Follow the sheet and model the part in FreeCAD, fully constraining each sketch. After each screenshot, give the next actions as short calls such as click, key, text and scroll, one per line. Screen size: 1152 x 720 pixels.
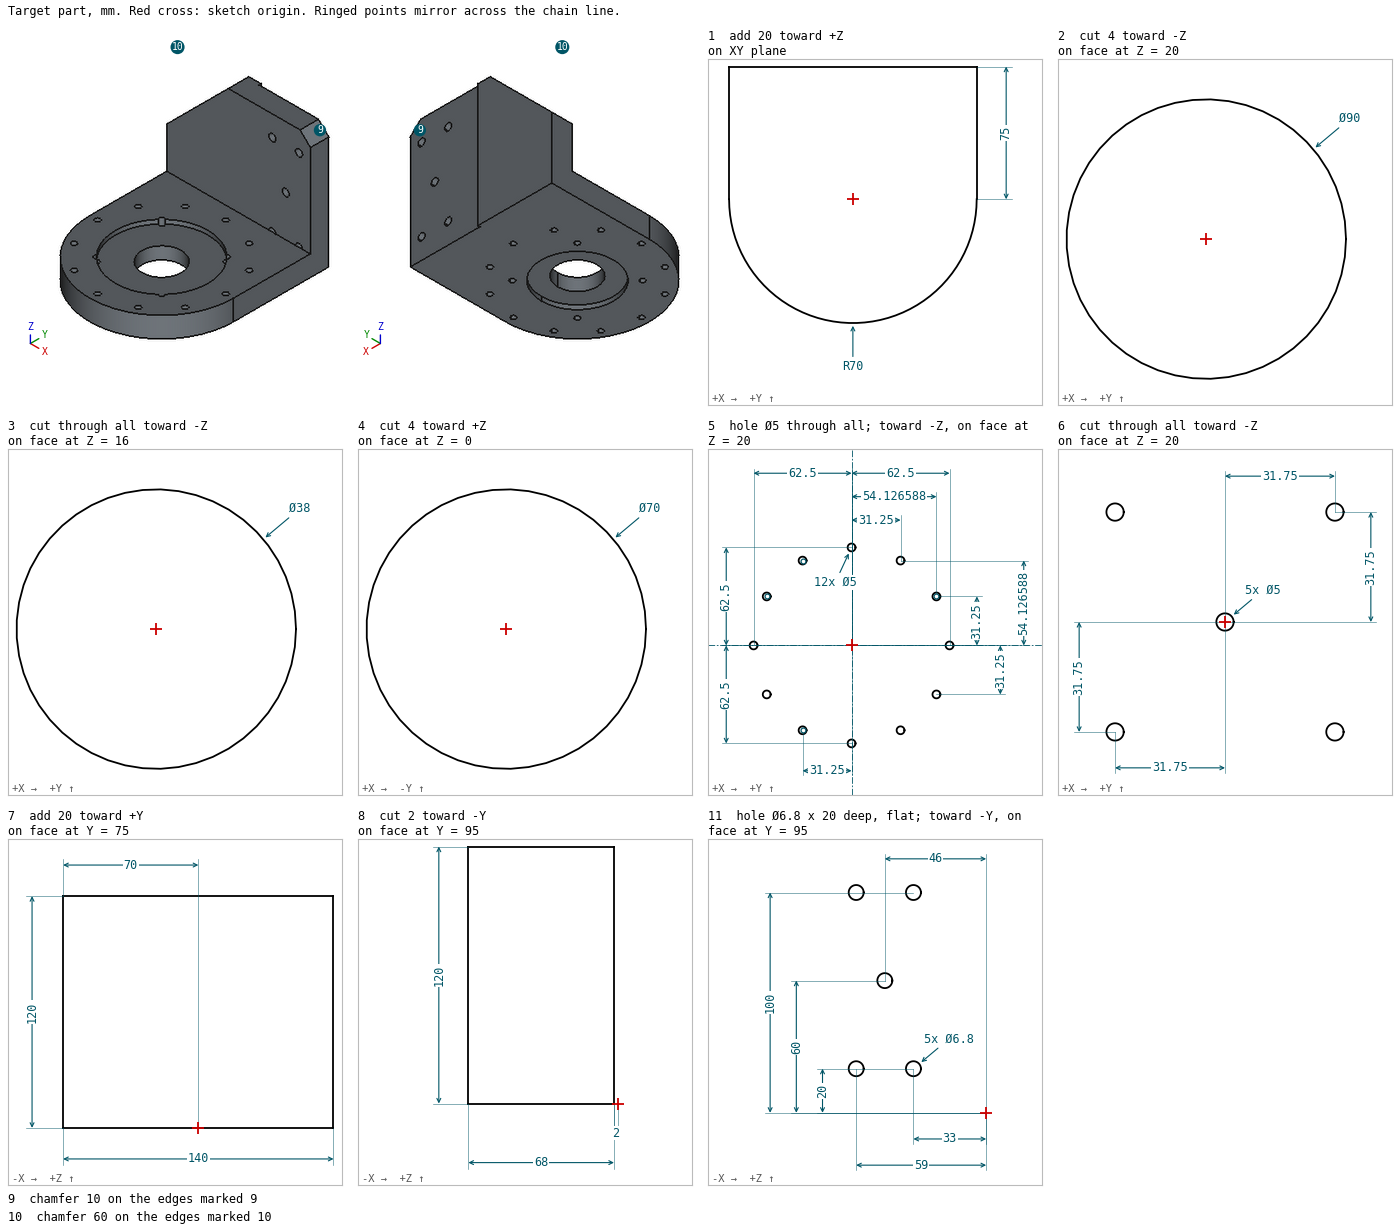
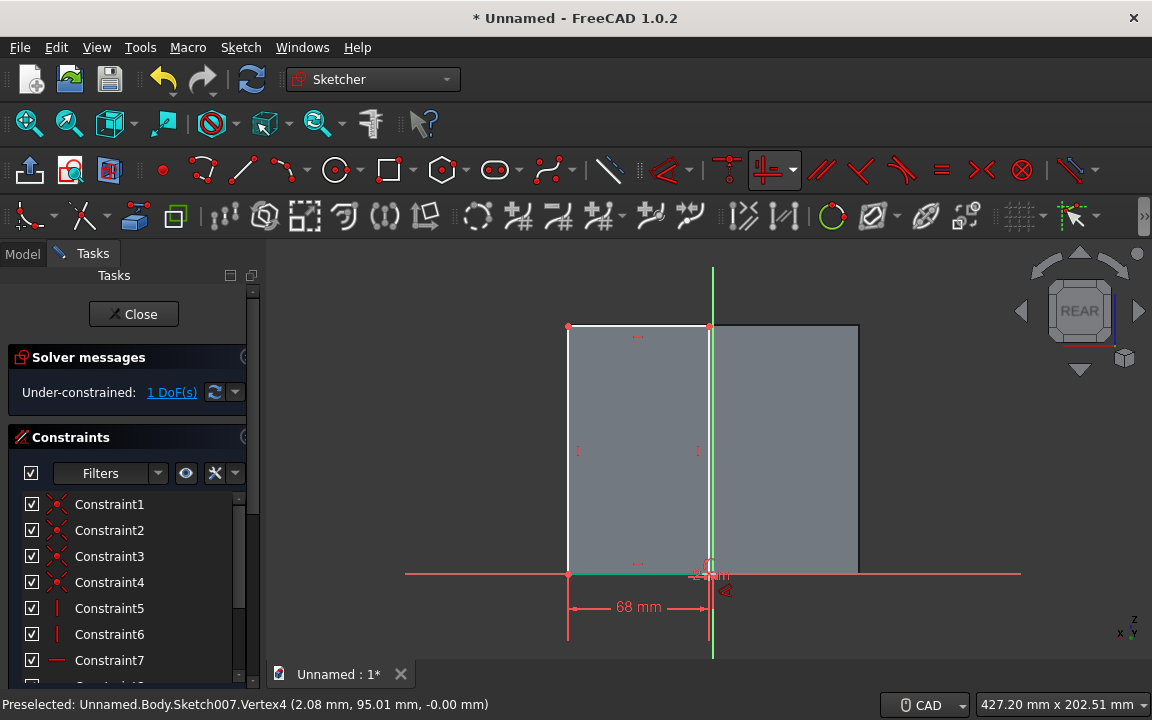
click(568, 401)
click(534, 450)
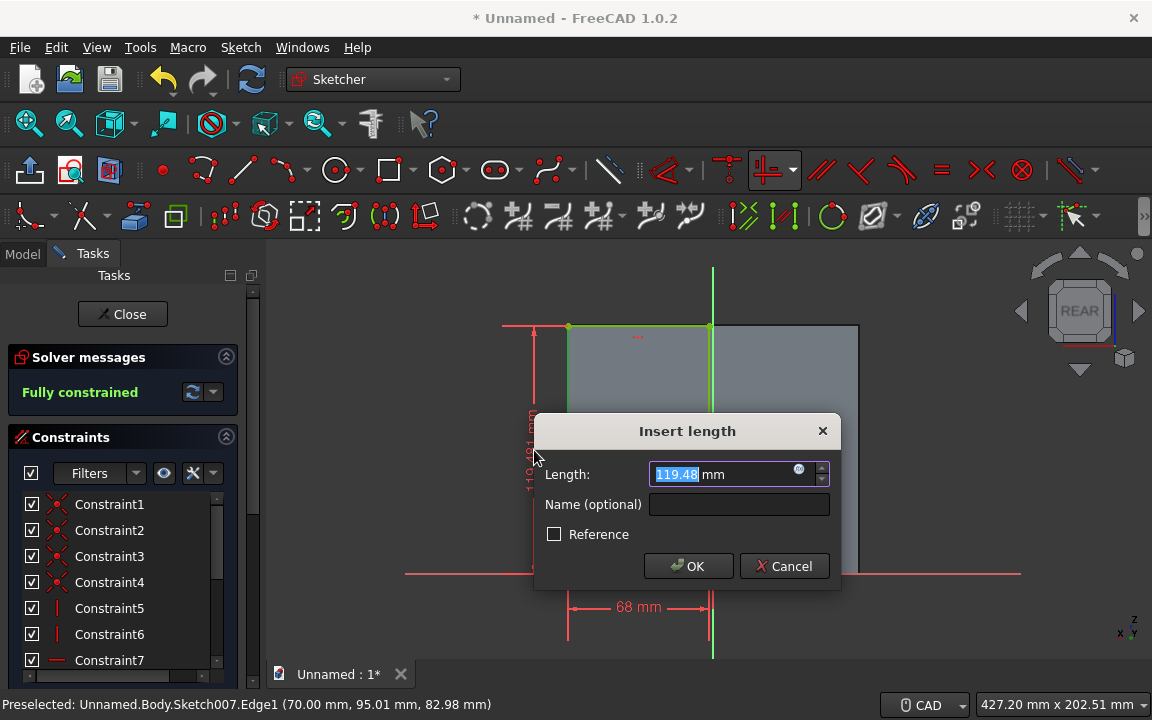
text(120)
key(Return)
key(Escape)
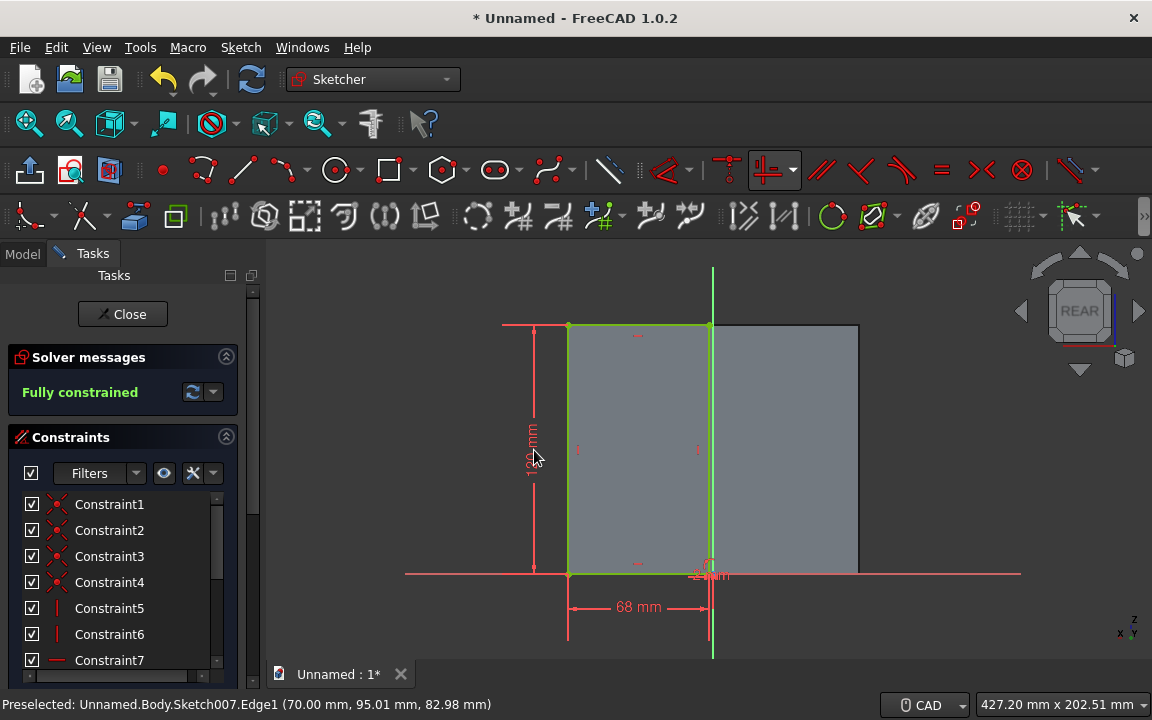
click(123, 314)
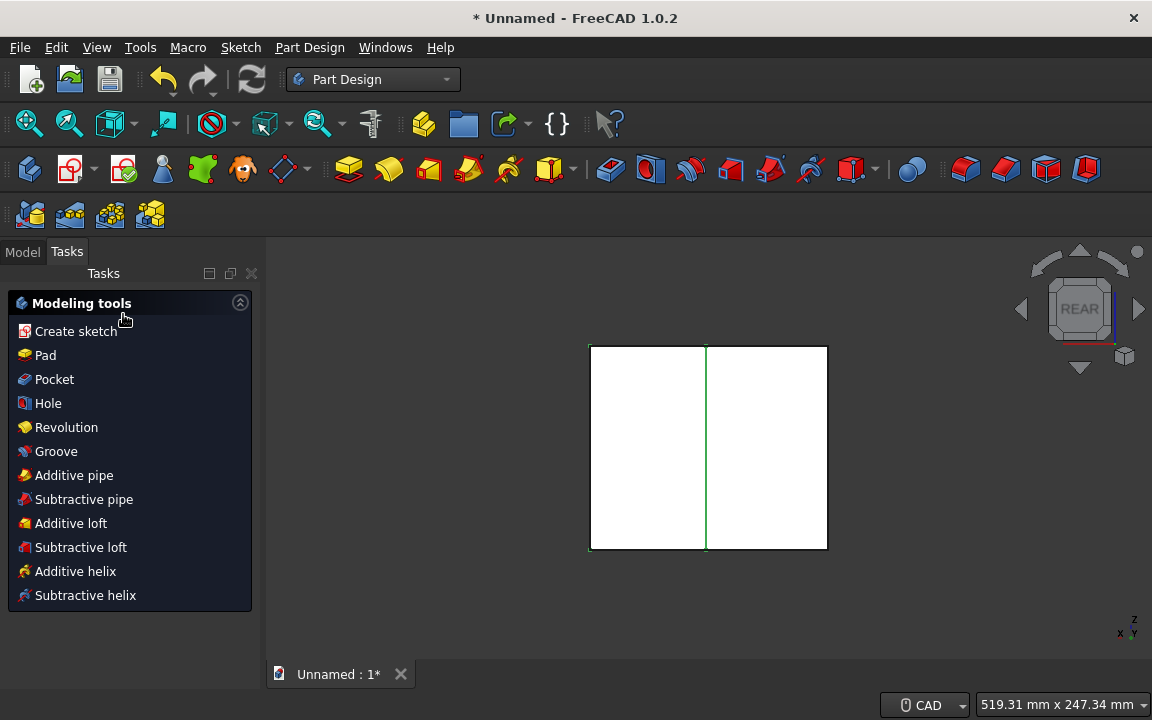
click(612, 170)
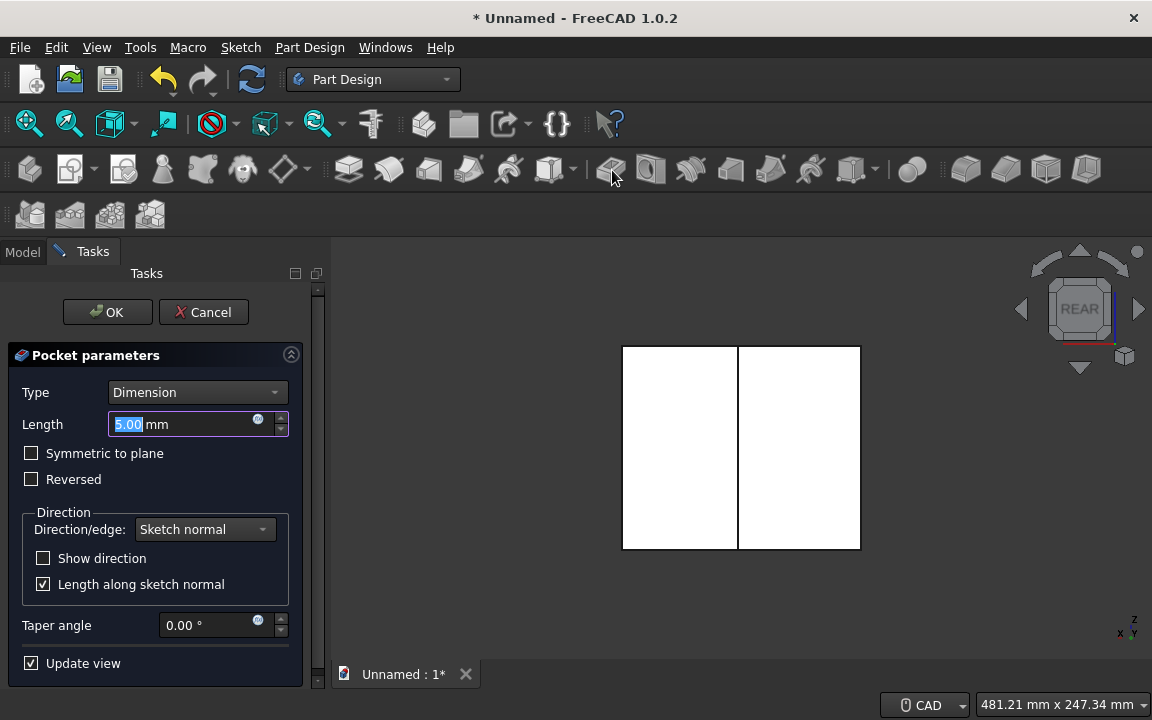
text(2)
key(Tab)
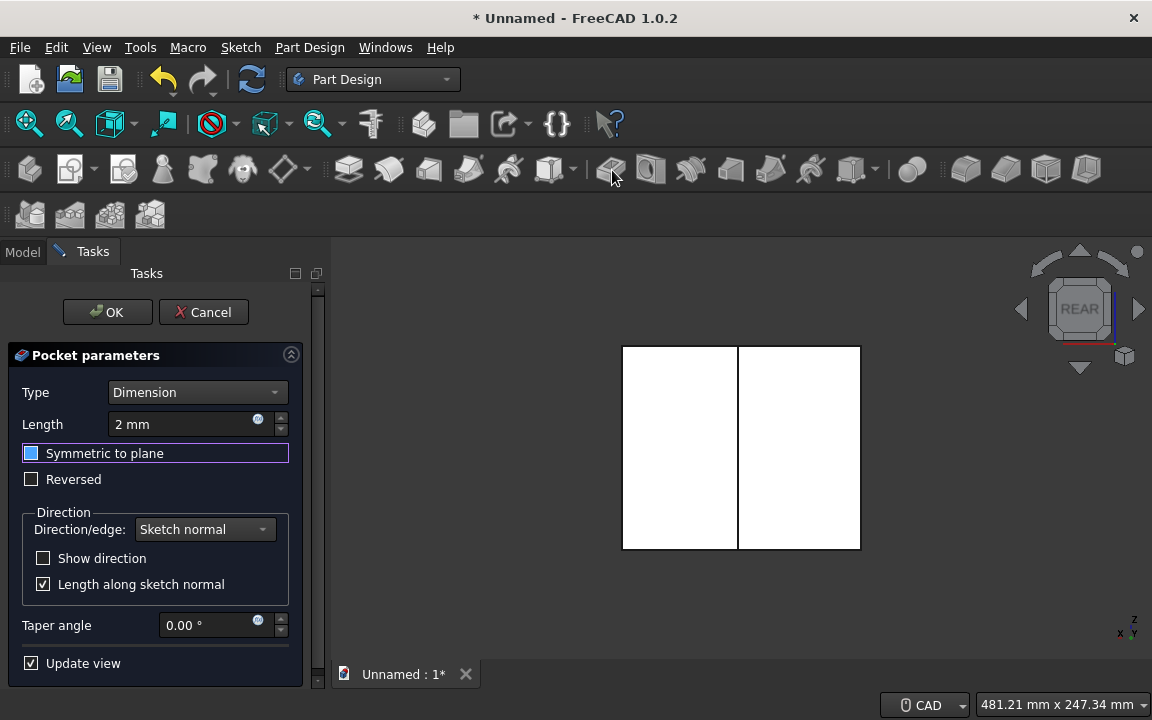
click(108, 312)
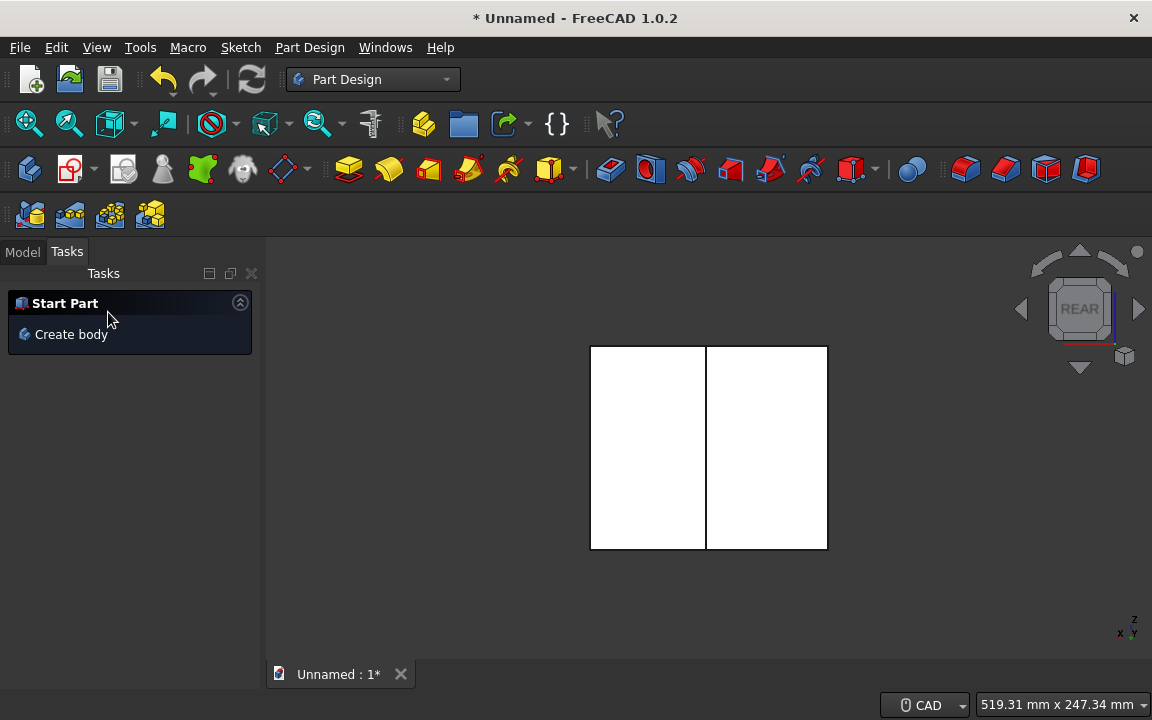
key(0)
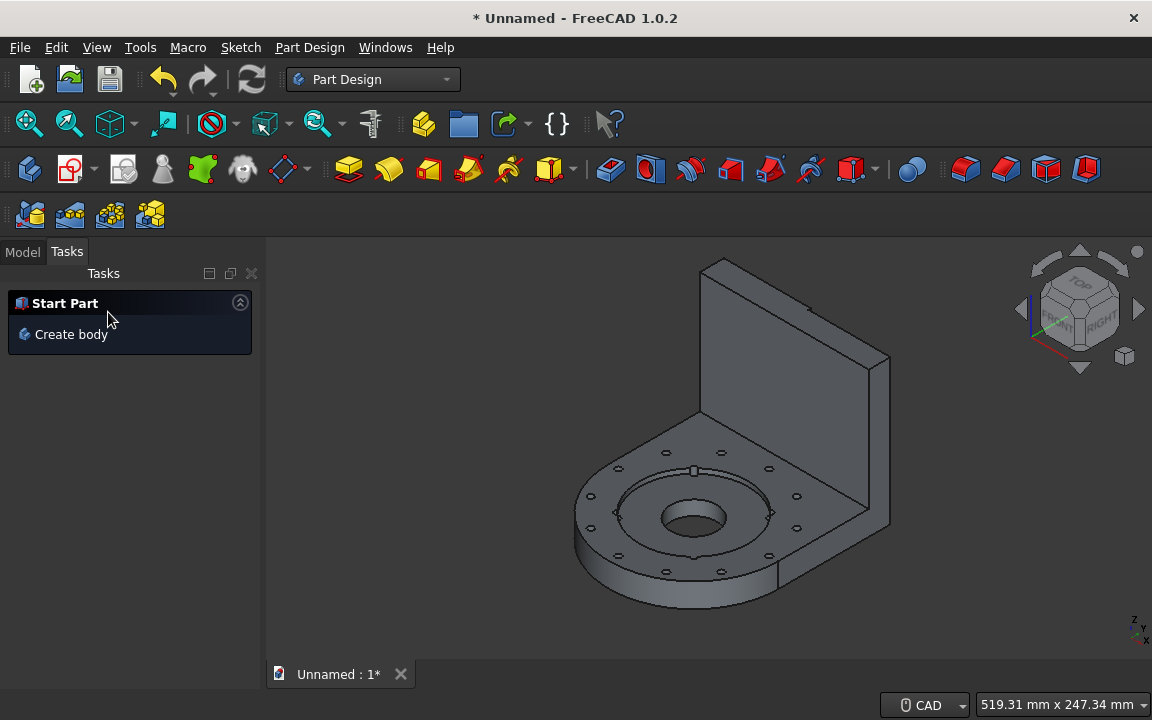
click(880, 362)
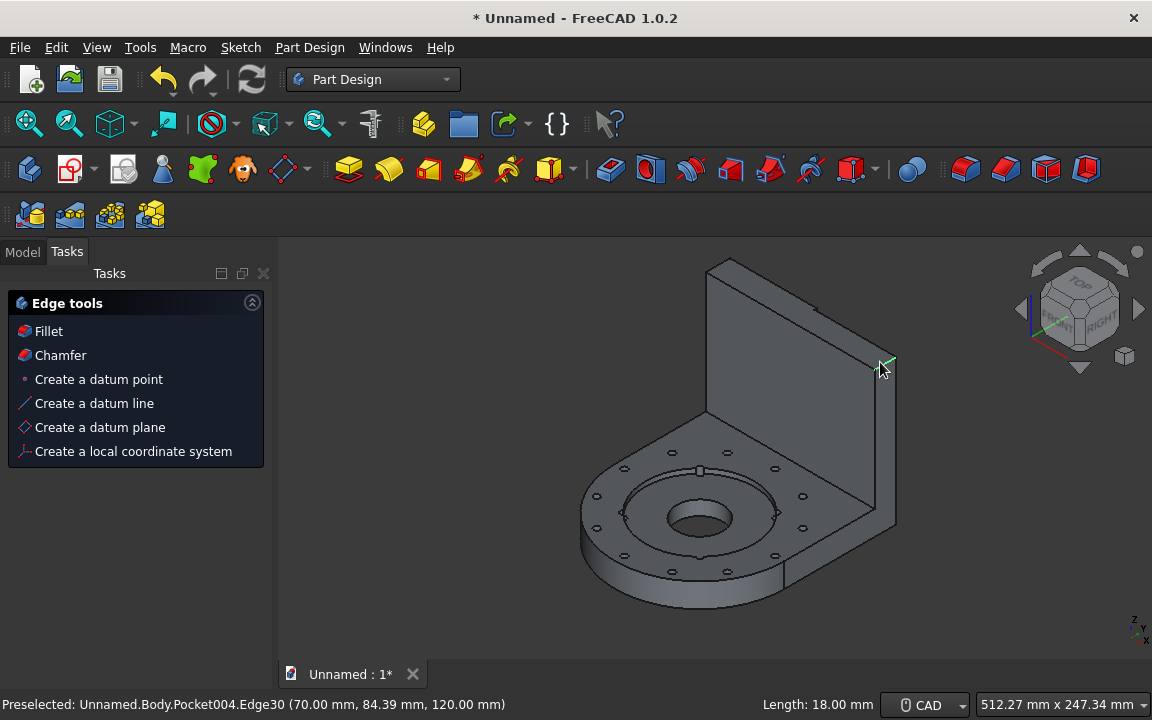
click(1006, 170)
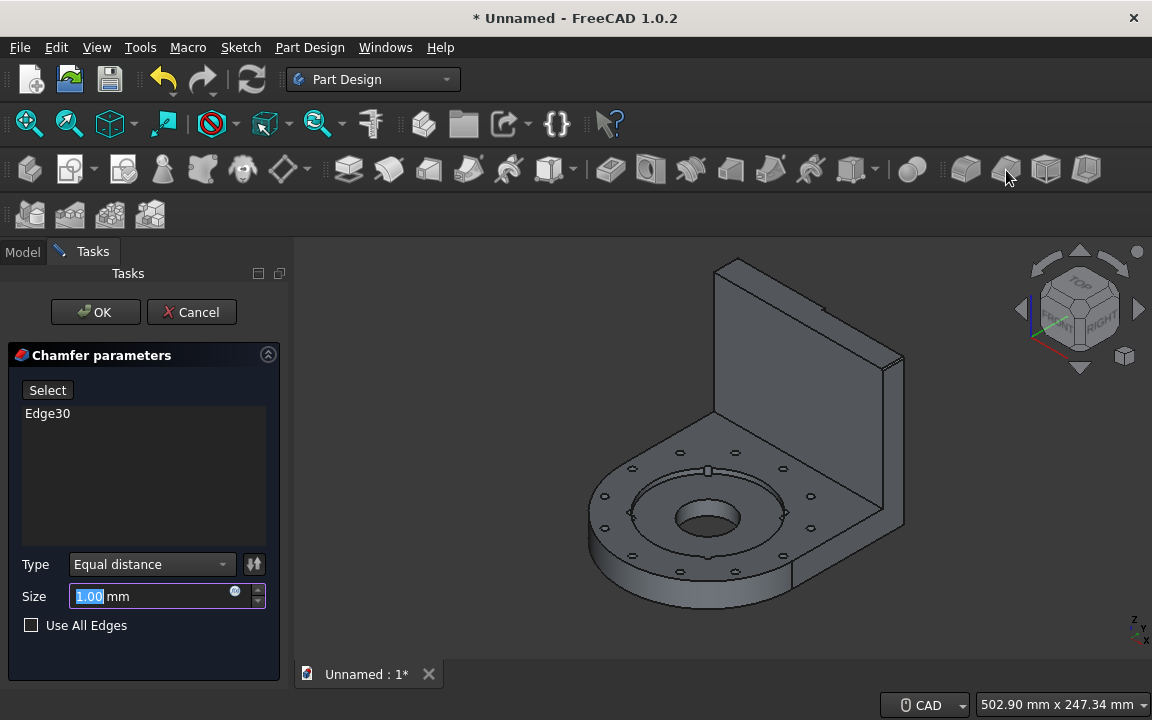
text(10)
key(Tab)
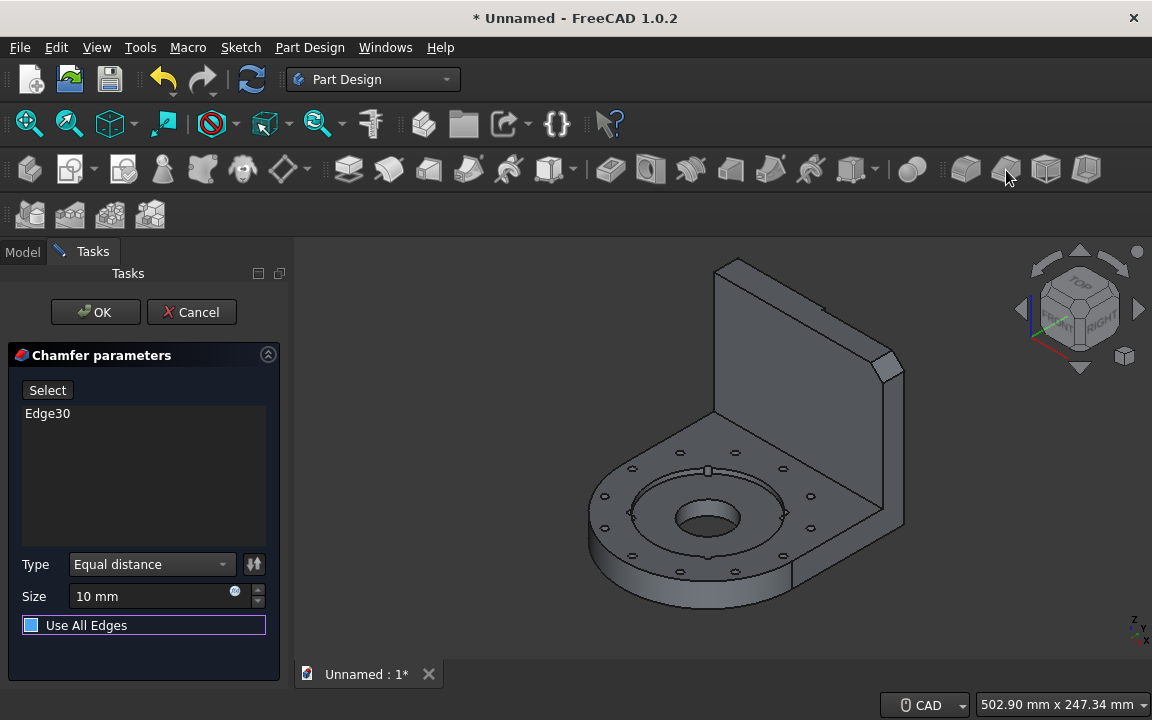
click(96, 312)